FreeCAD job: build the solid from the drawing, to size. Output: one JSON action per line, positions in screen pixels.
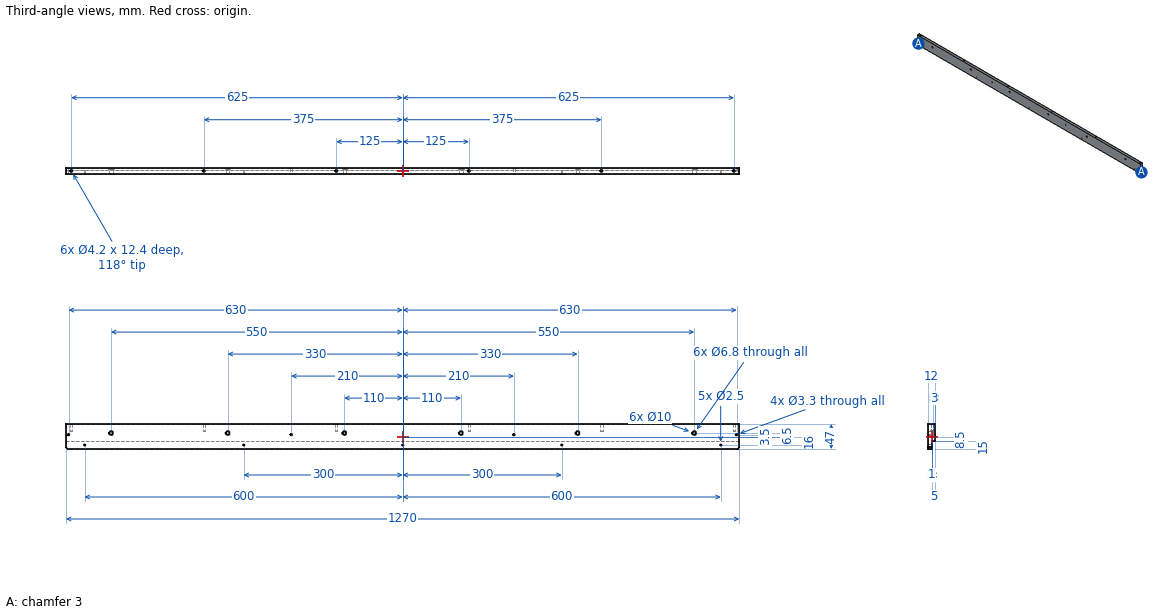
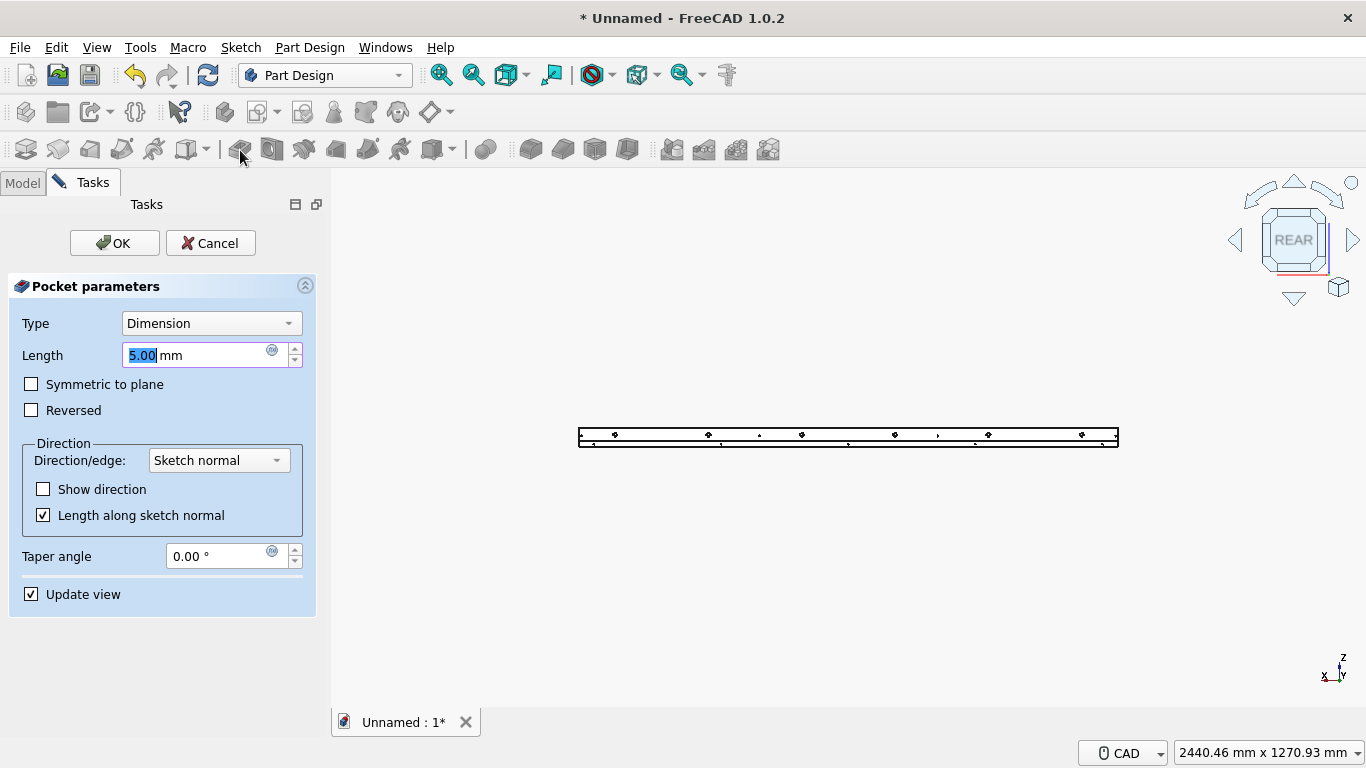
{"action": "type", "text": "3"}
{"action": "key", "text": "Tab"}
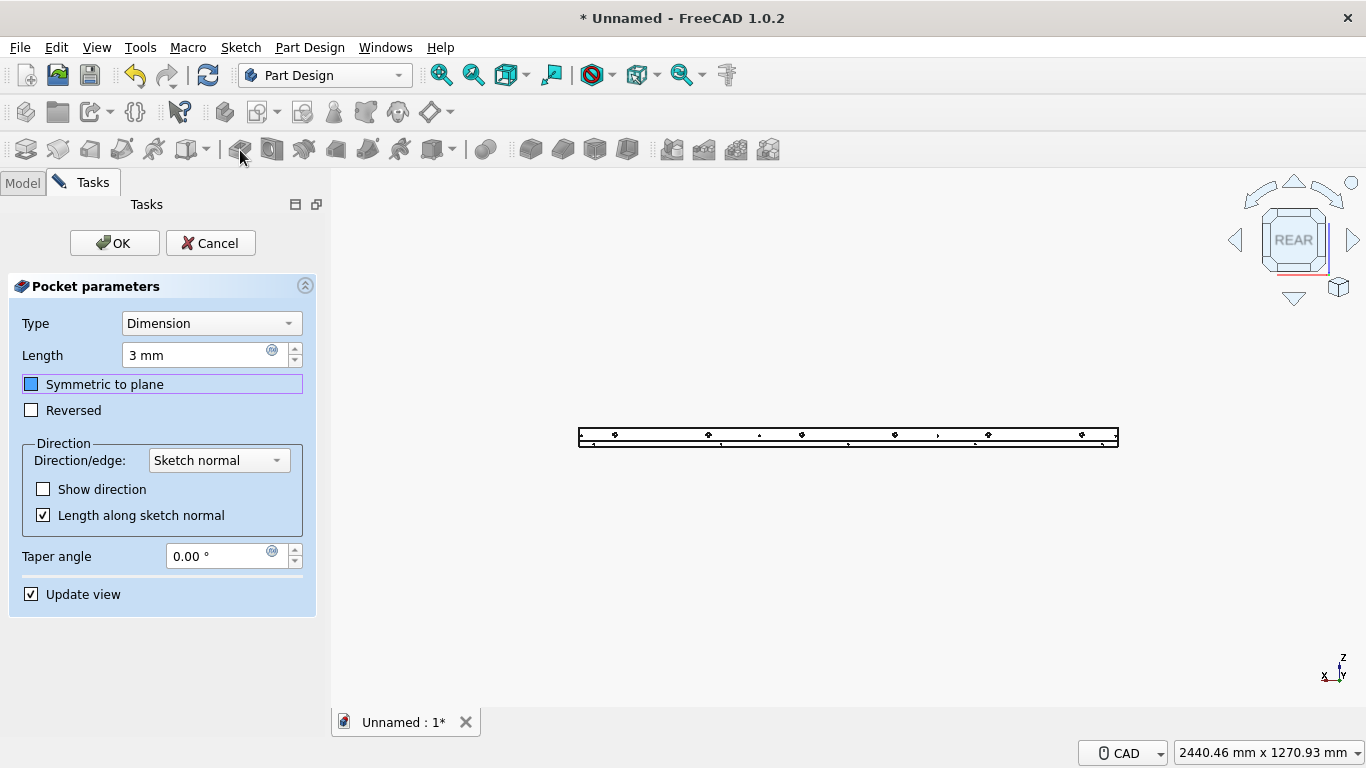
{"action": "left_click", "coordinate": [115, 243]}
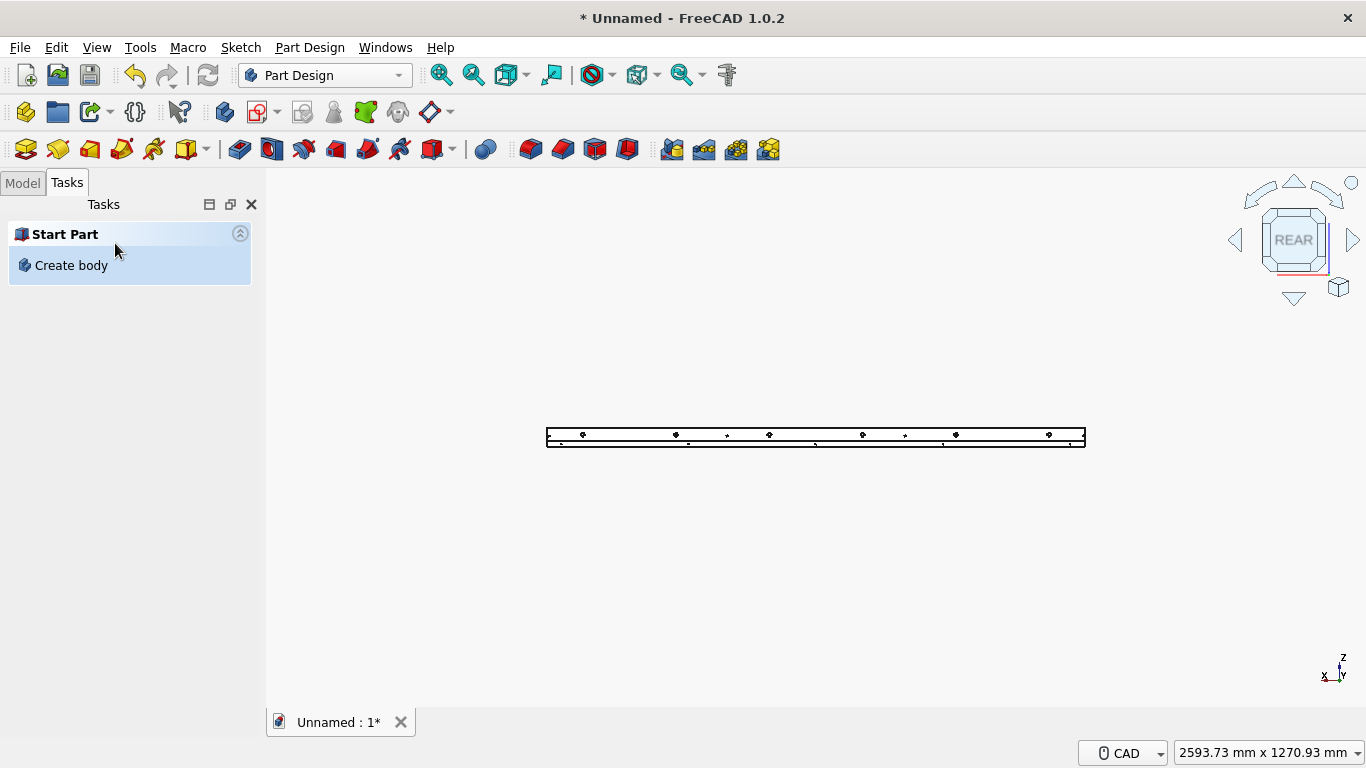
{"action": "key", "text": "0"}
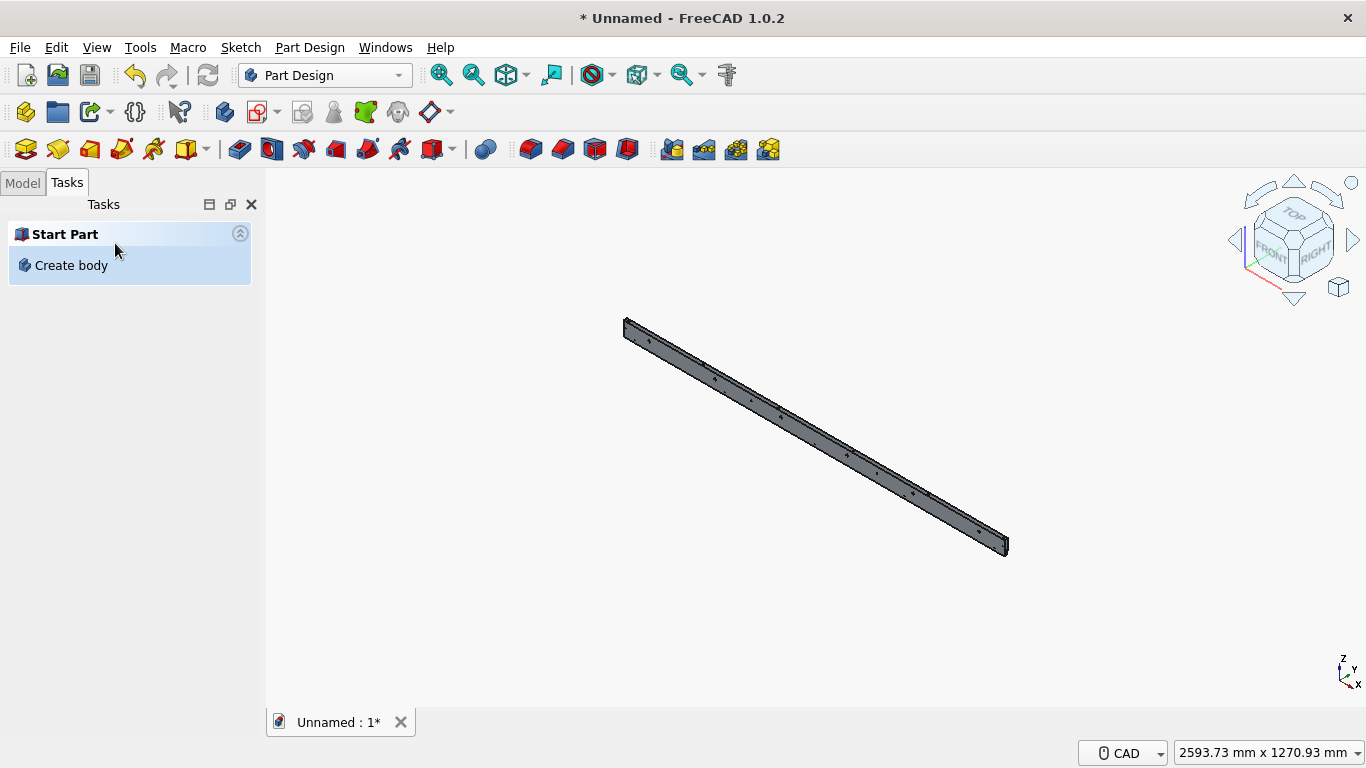
{"action": "left_click", "coordinate": [442, 76]}